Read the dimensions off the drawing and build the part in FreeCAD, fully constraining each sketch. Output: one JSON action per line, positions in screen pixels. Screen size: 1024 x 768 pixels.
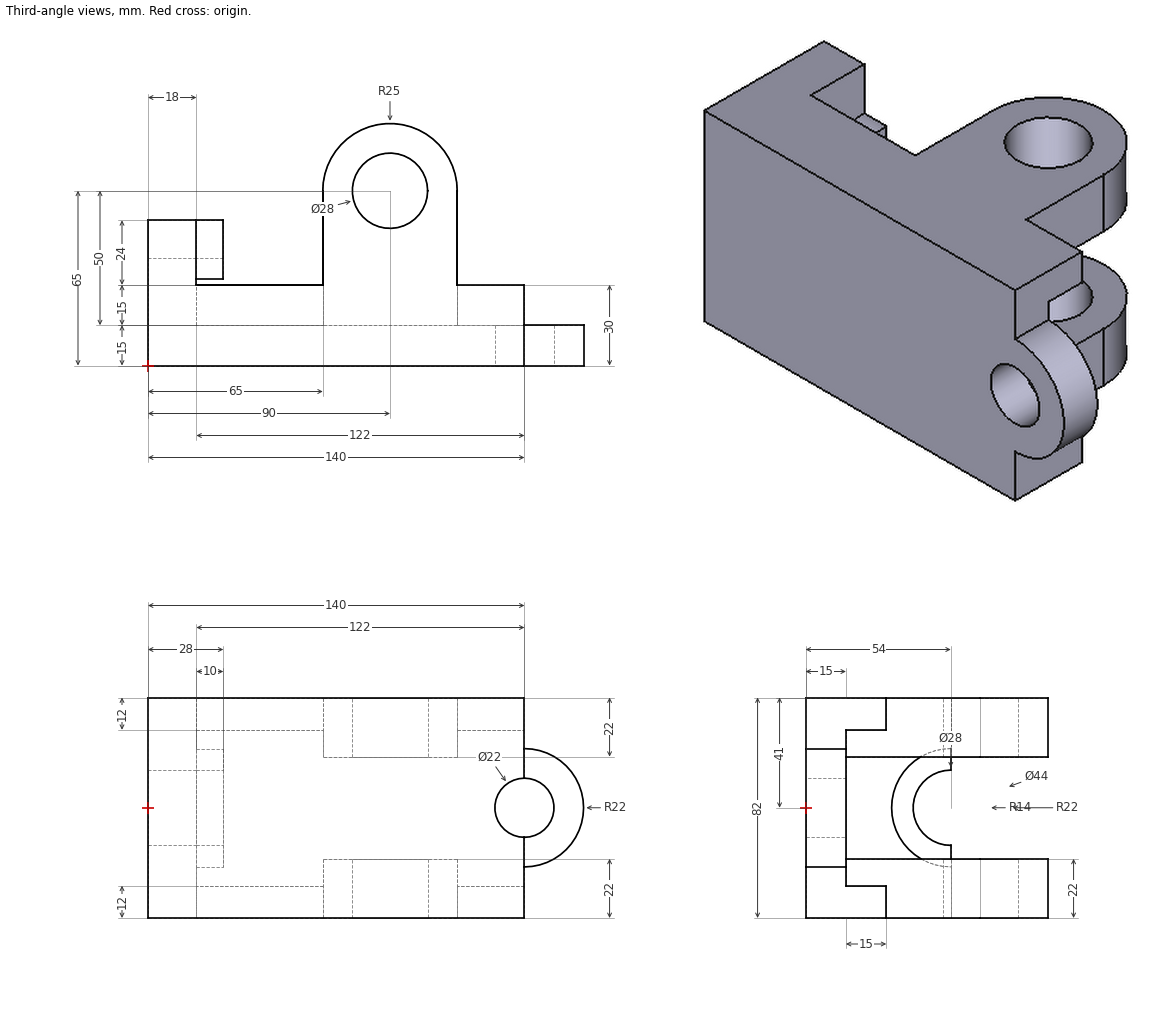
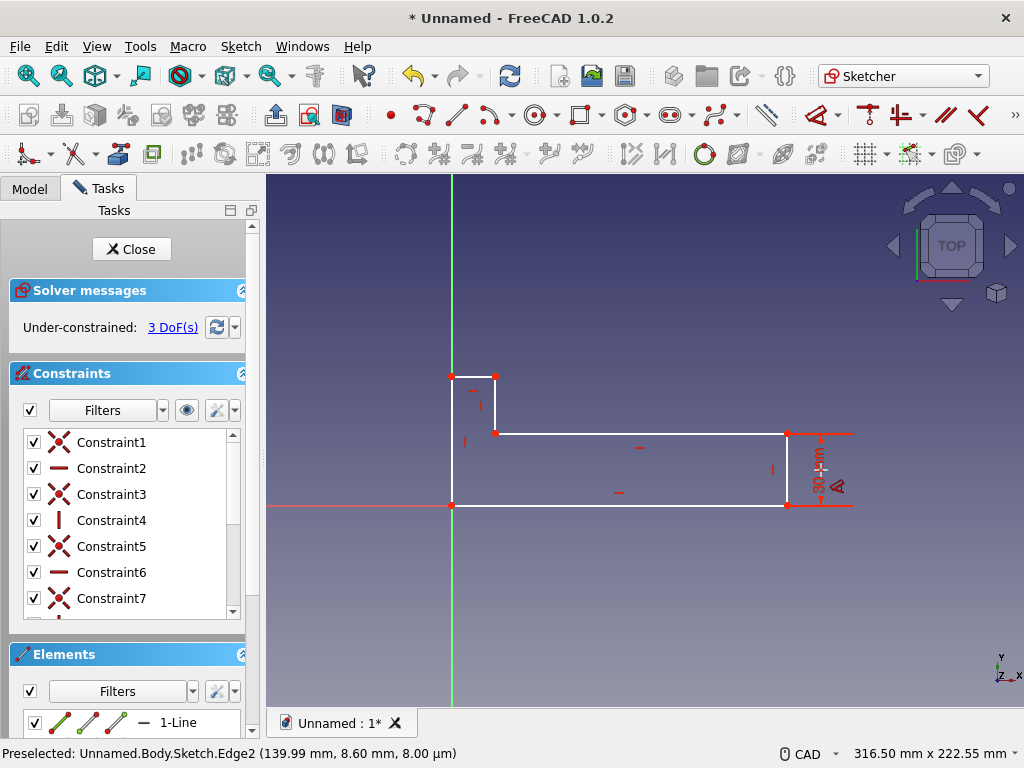
{"action": "left_click", "coordinate": [495, 417]}
{"action": "left_click", "coordinate": [529, 405]}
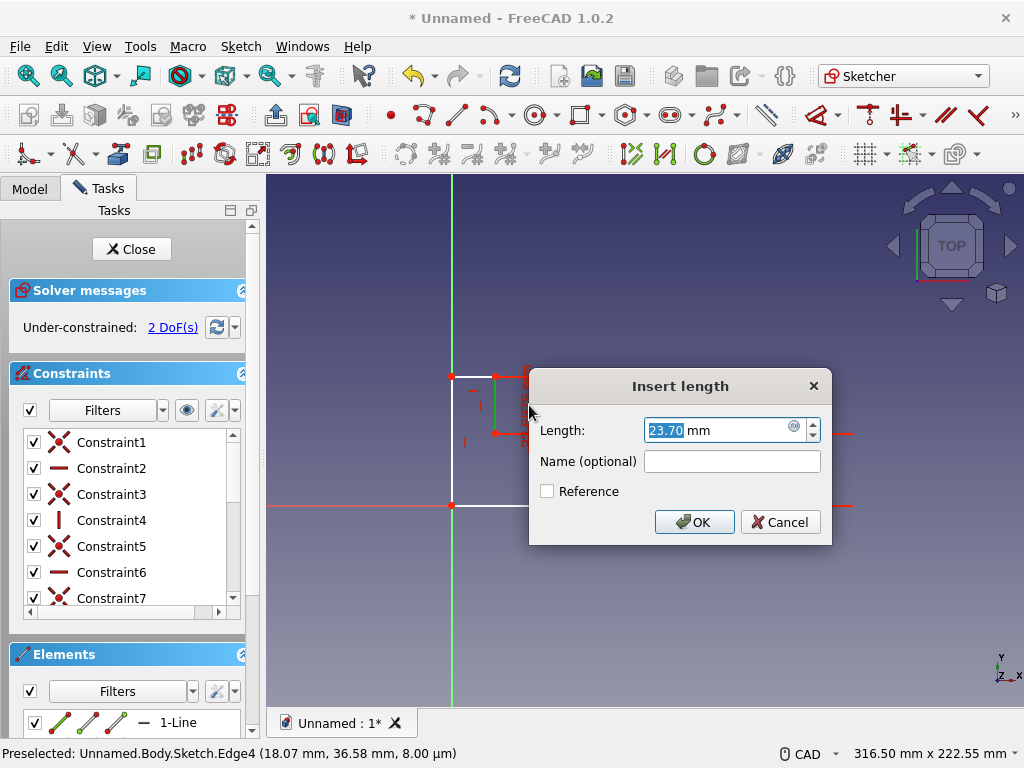
{"action": "type", "text": "24"}
{"action": "key", "text": "Return"}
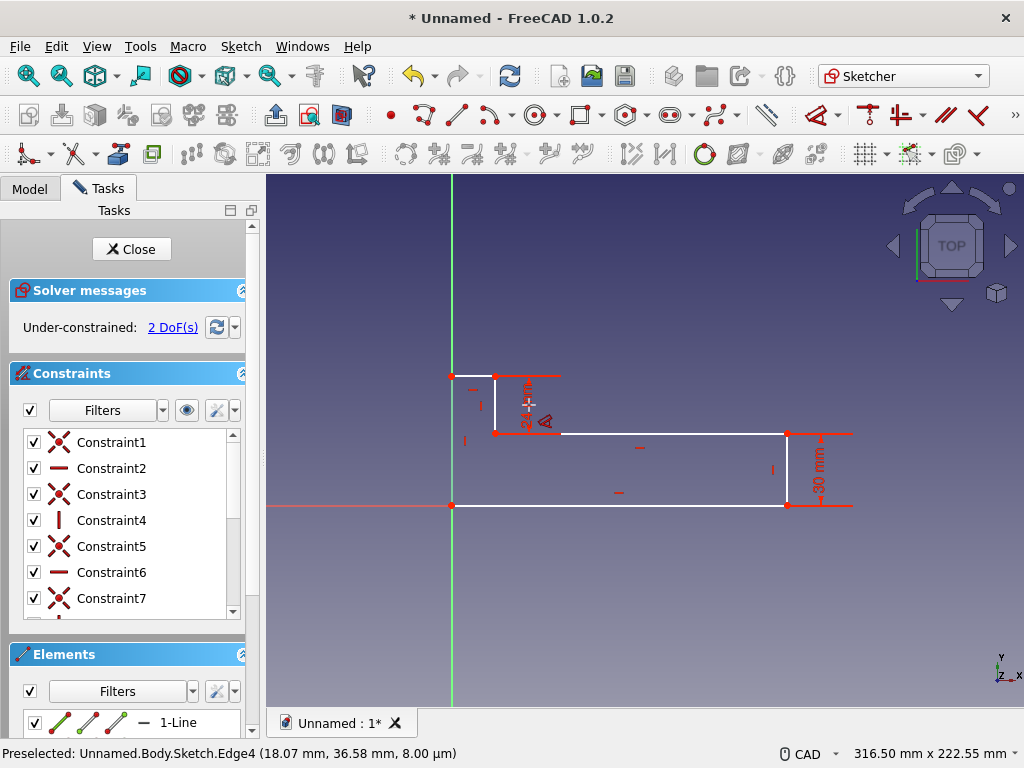
{"action": "left_click", "coordinate": [482, 376]}
{"action": "left_click", "coordinate": [473, 342]}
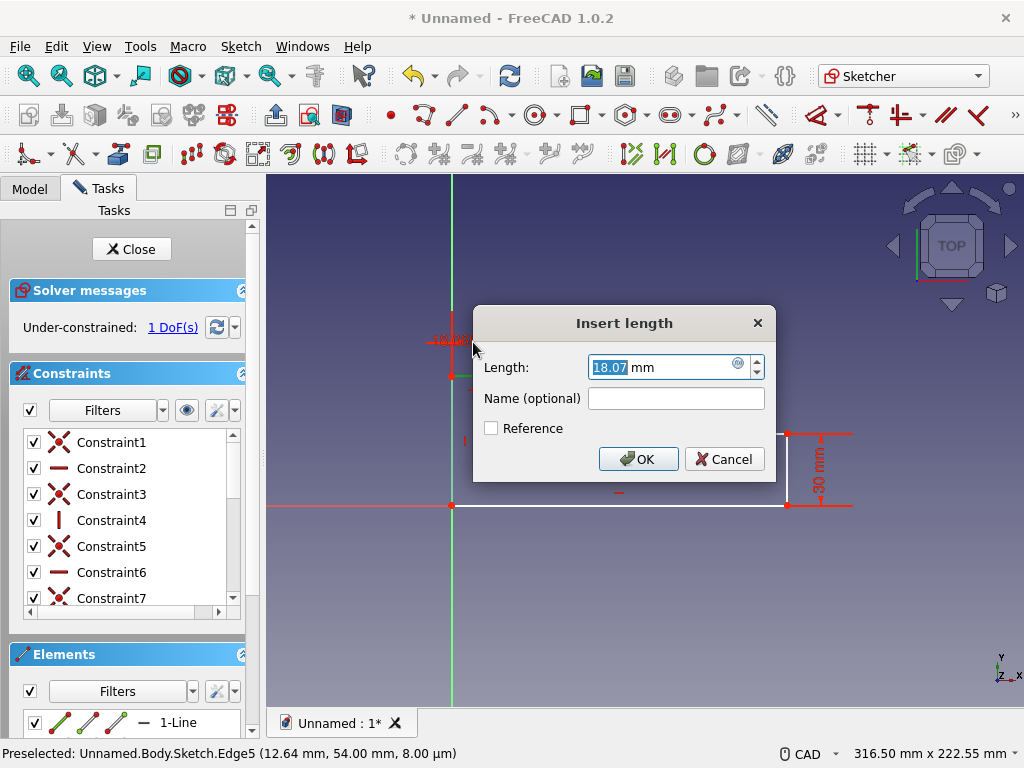
{"action": "type", "text": "18"}
{"action": "key", "text": "Return"}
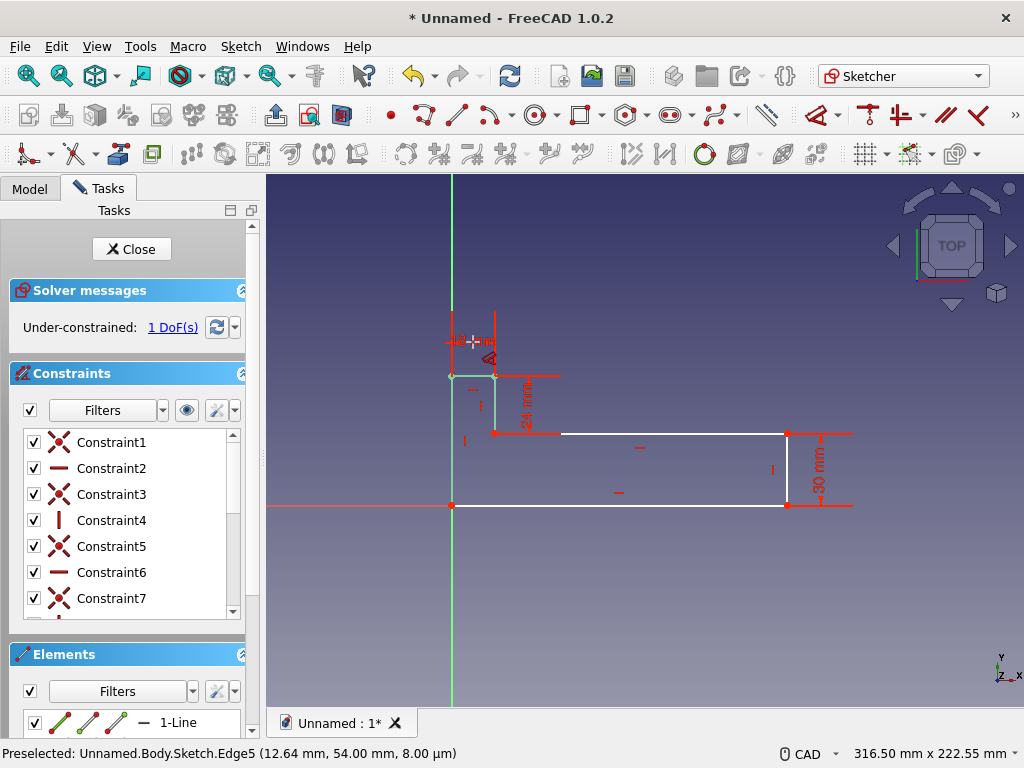
{"action": "left_click", "coordinate": [552, 506]}
{"action": "left_click", "coordinate": [619, 540]}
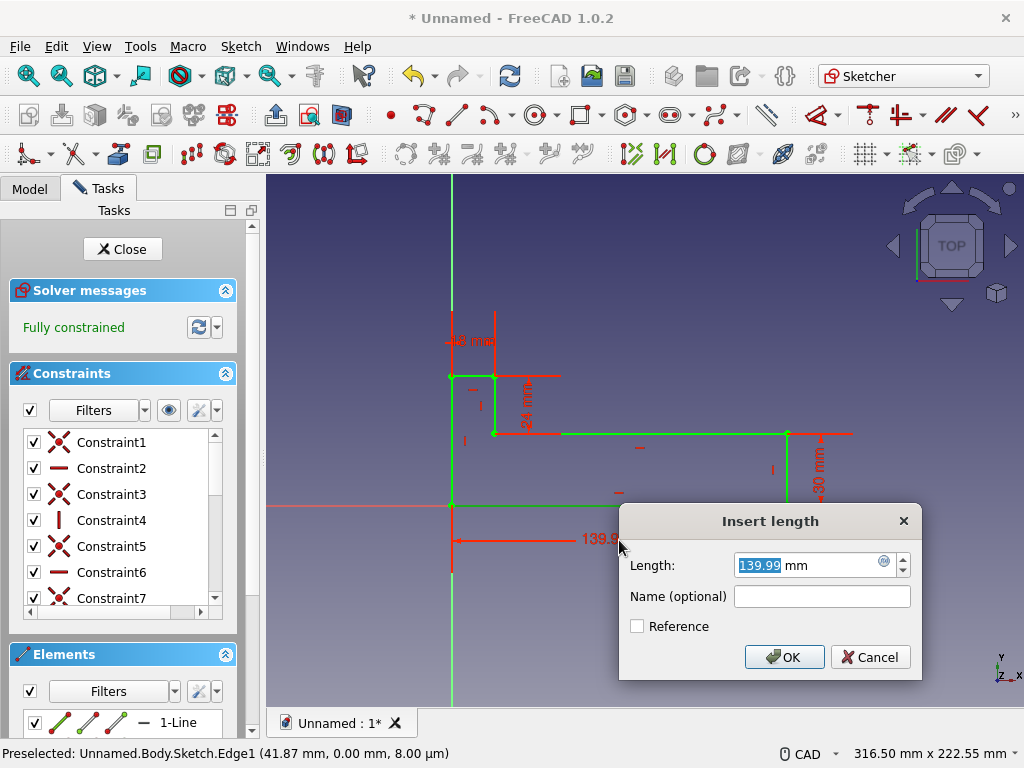
{"action": "type", "text": "140"}
{"action": "key", "text": "Return"}
{"action": "key", "text": "Escape"}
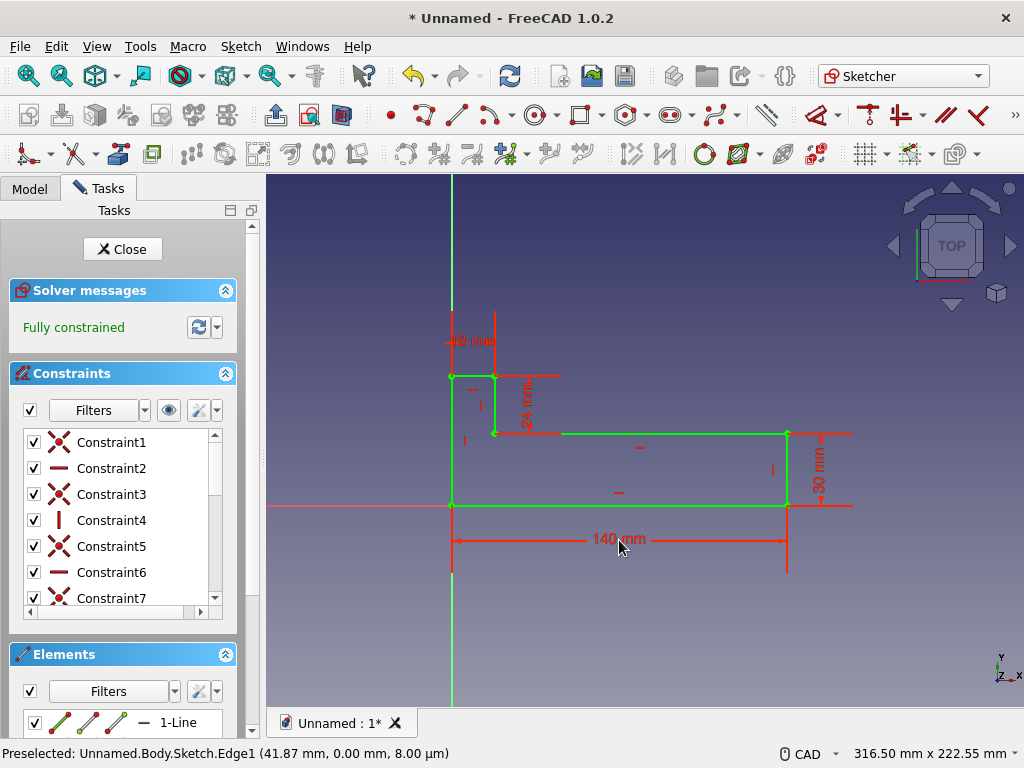
{"action": "left_click", "coordinate": [123, 249]}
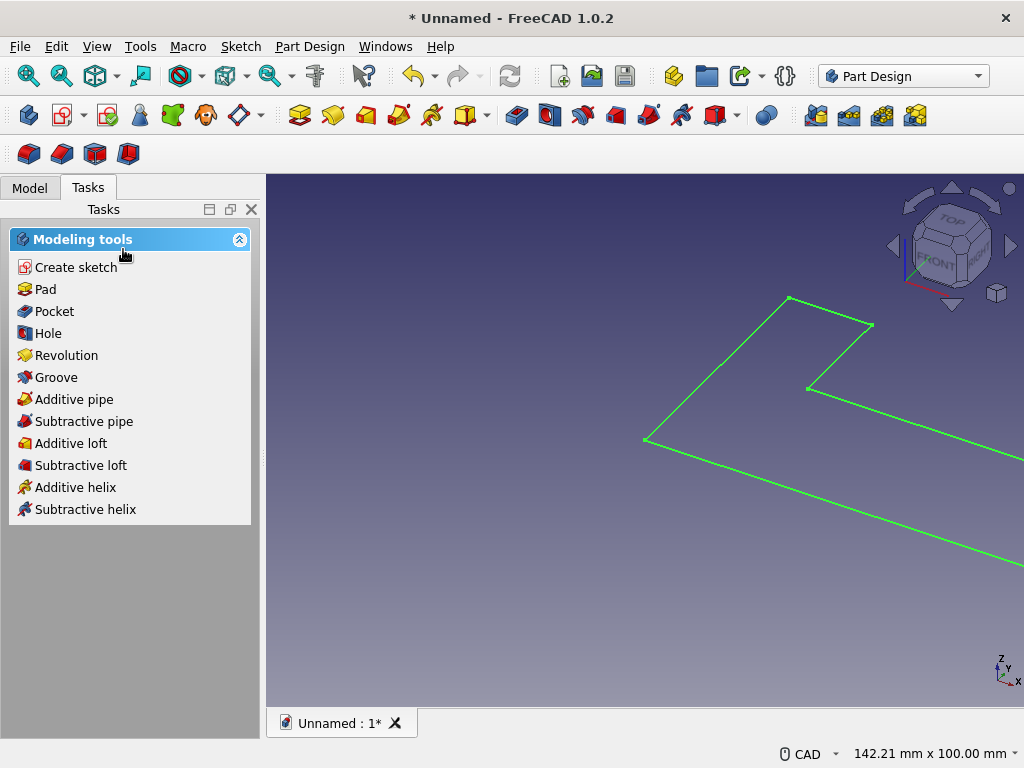
{"action": "left_click", "coordinate": [300, 116]}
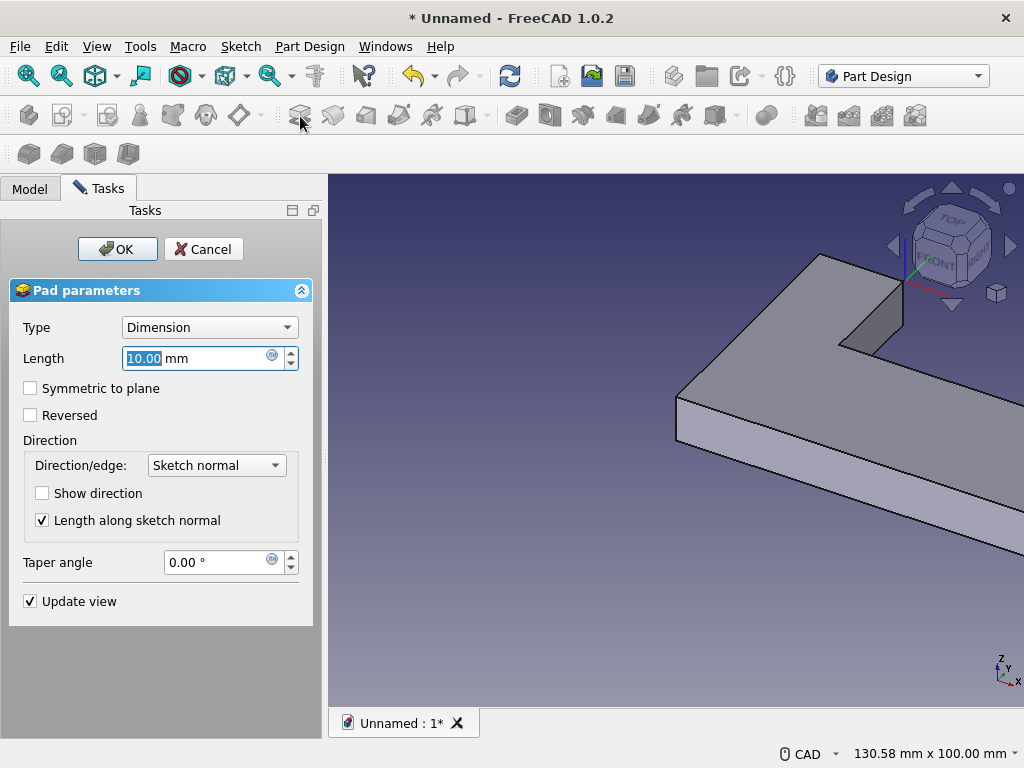
{"action": "type", "text": "82"}
{"action": "key", "text": "Tab"}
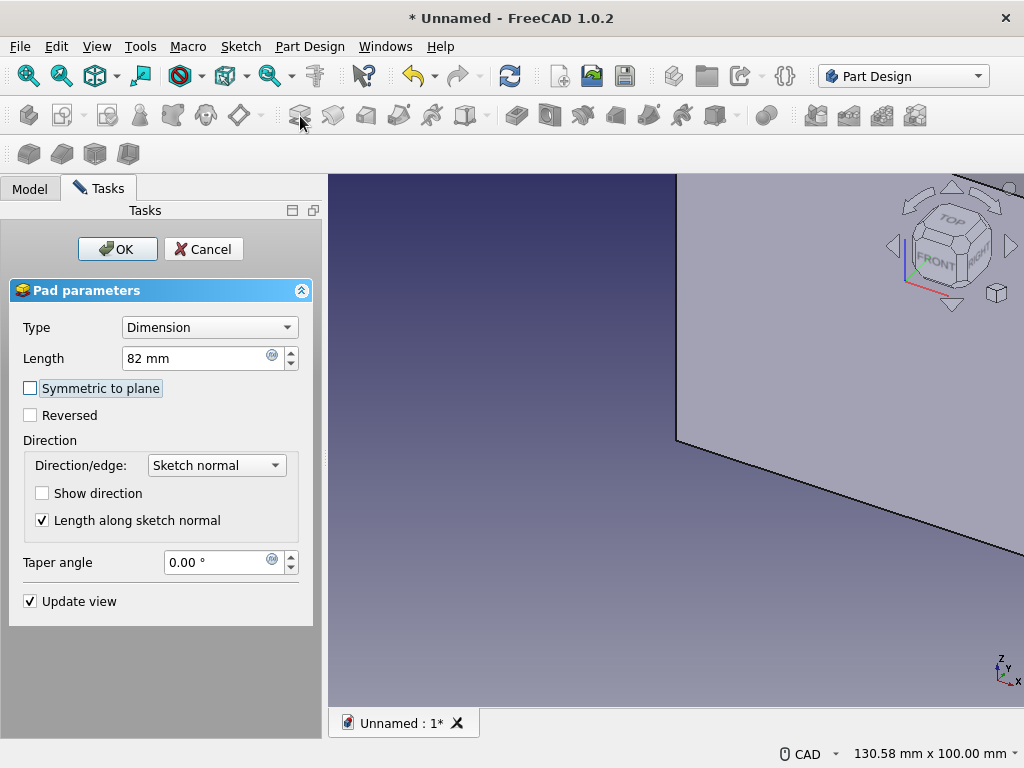
{"action": "left_click", "coordinate": [31, 388]}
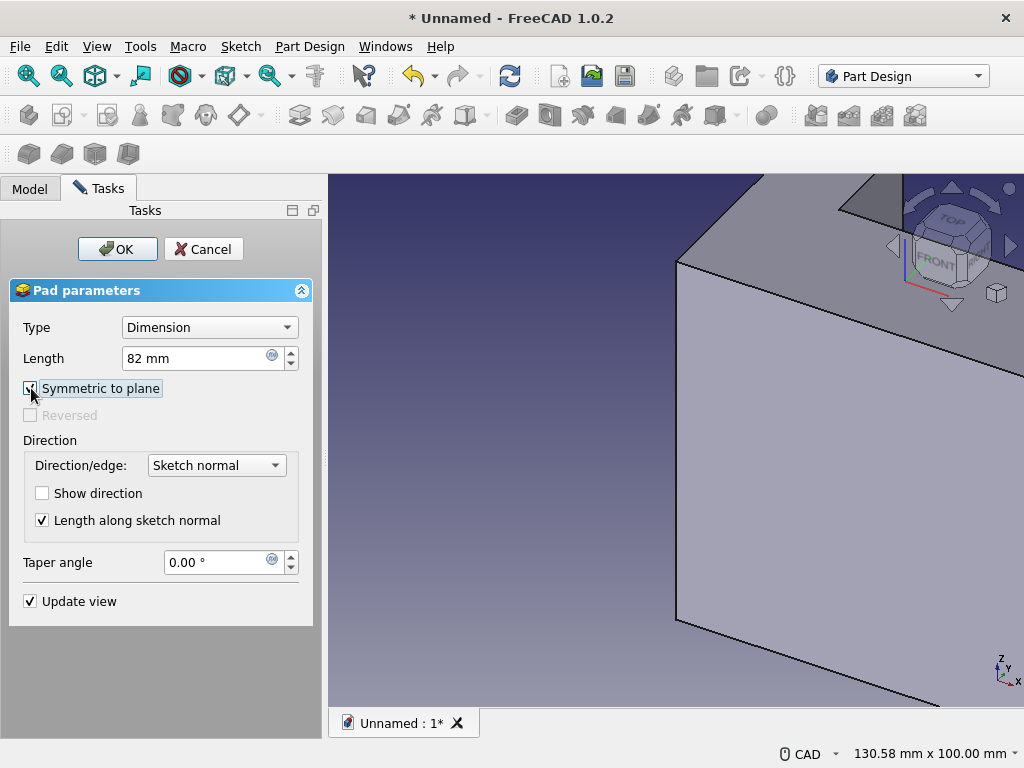
{"action": "left_click", "coordinate": [118, 249]}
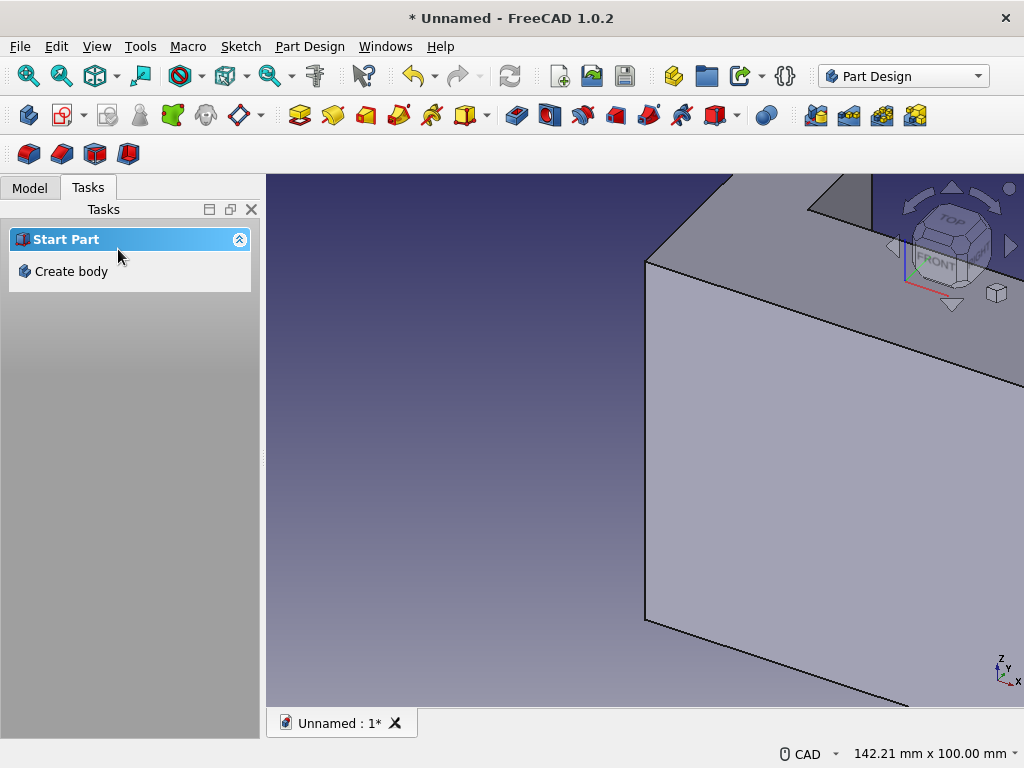
{"action": "left_click", "coordinate": [29, 76]}